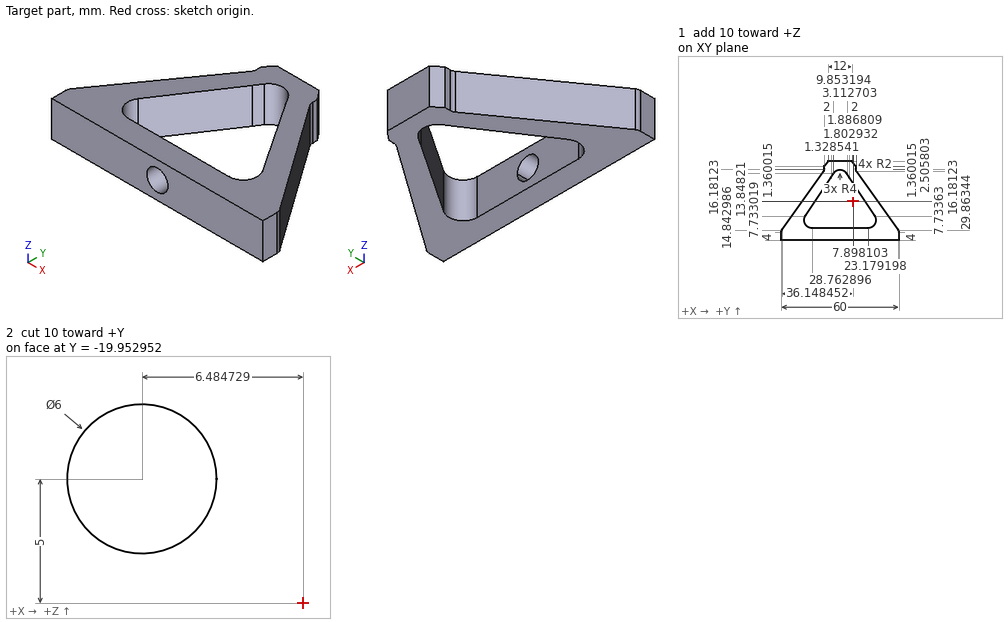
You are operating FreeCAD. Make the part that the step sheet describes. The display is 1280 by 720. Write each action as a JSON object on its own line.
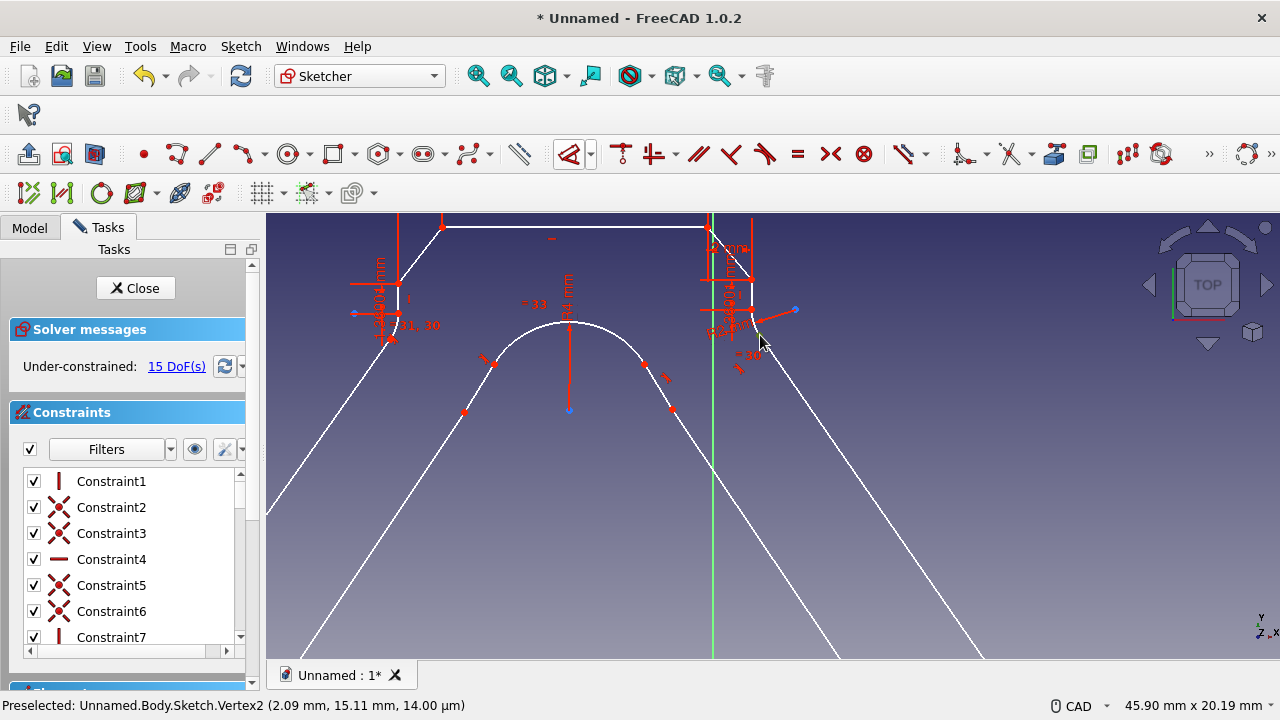
{"action": "left_click", "coordinate": [590, 154]}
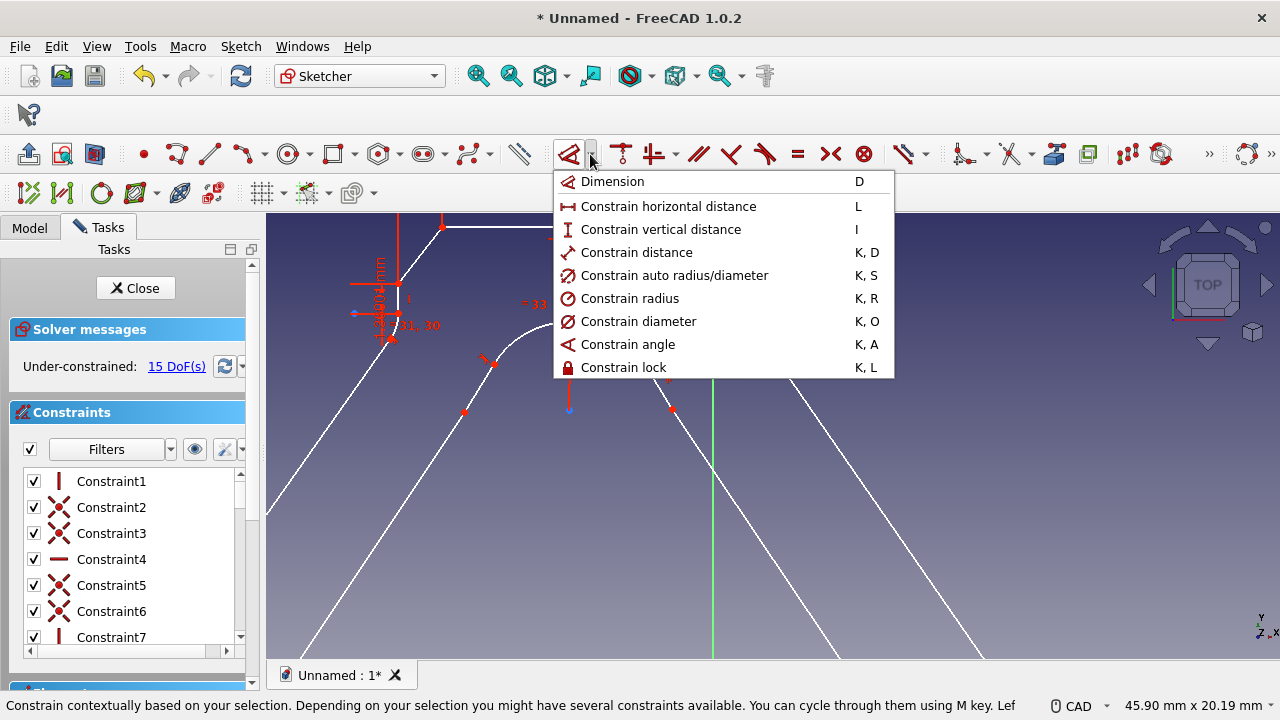
{"action": "left_click", "coordinate": [724, 206]}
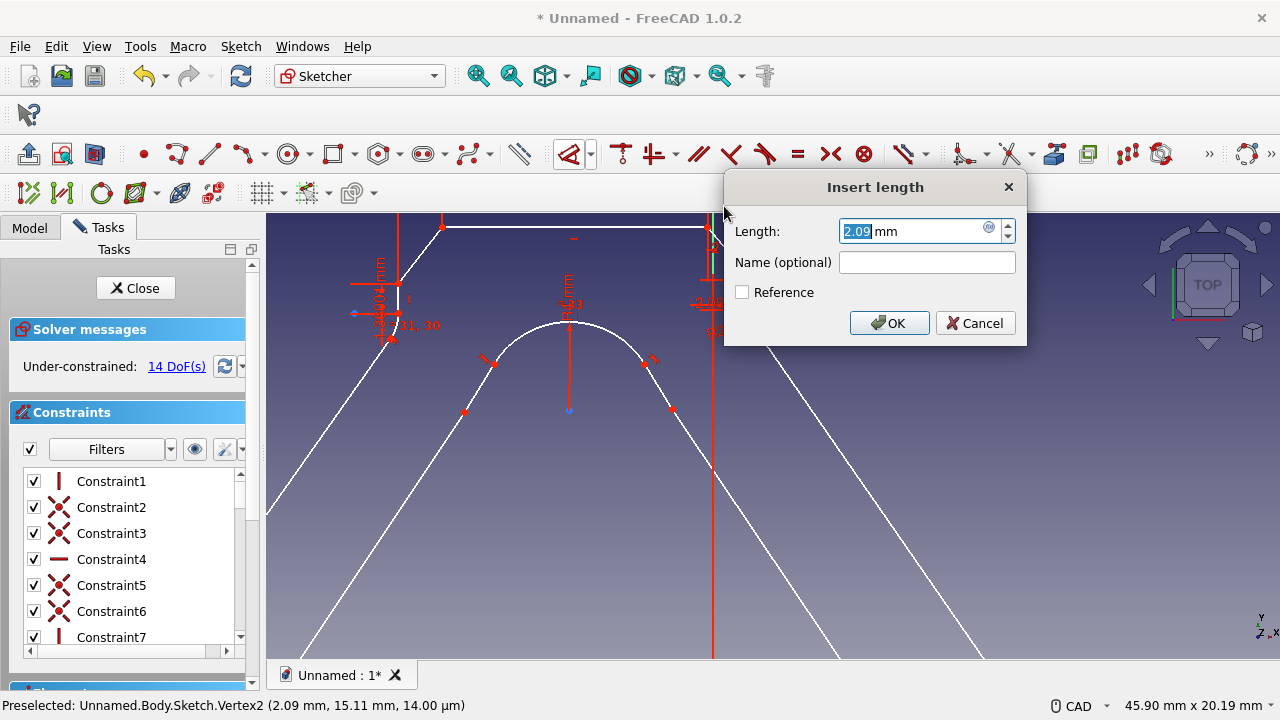
{"action": "type", "text": "1.886809"}
{"action": "key", "text": "Return"}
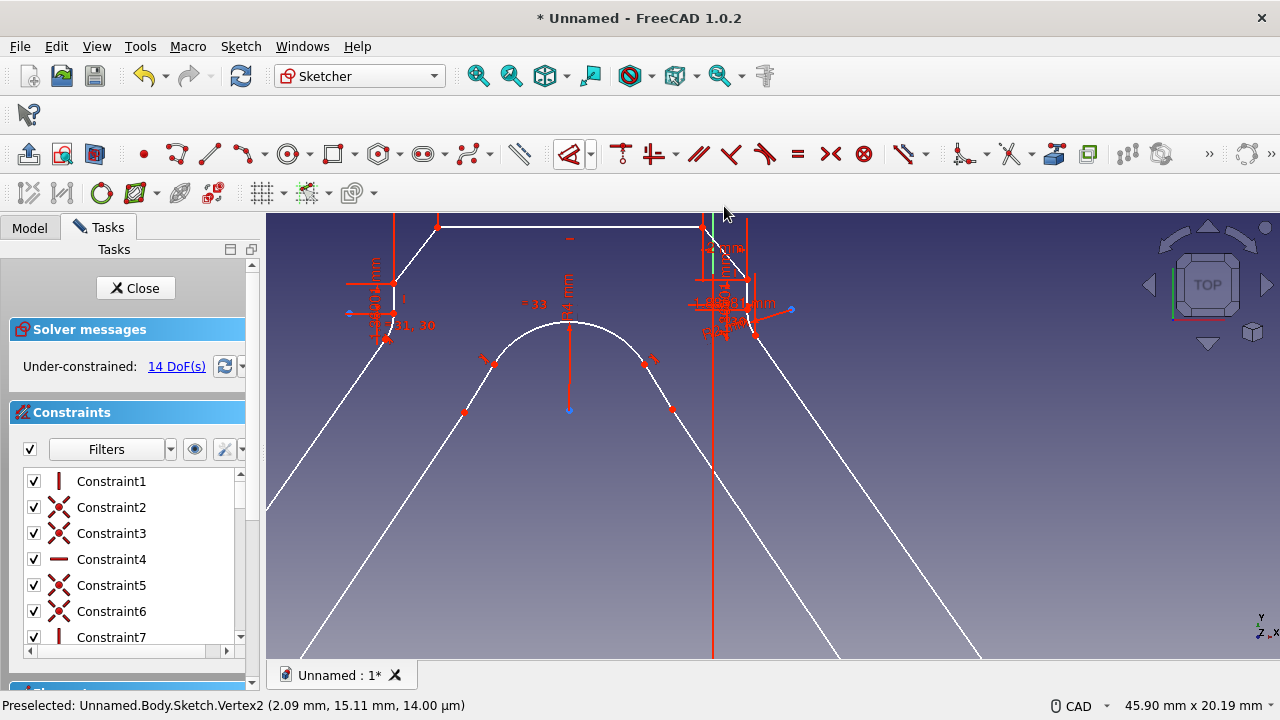
{"action": "left_click", "coordinate": [747, 310]}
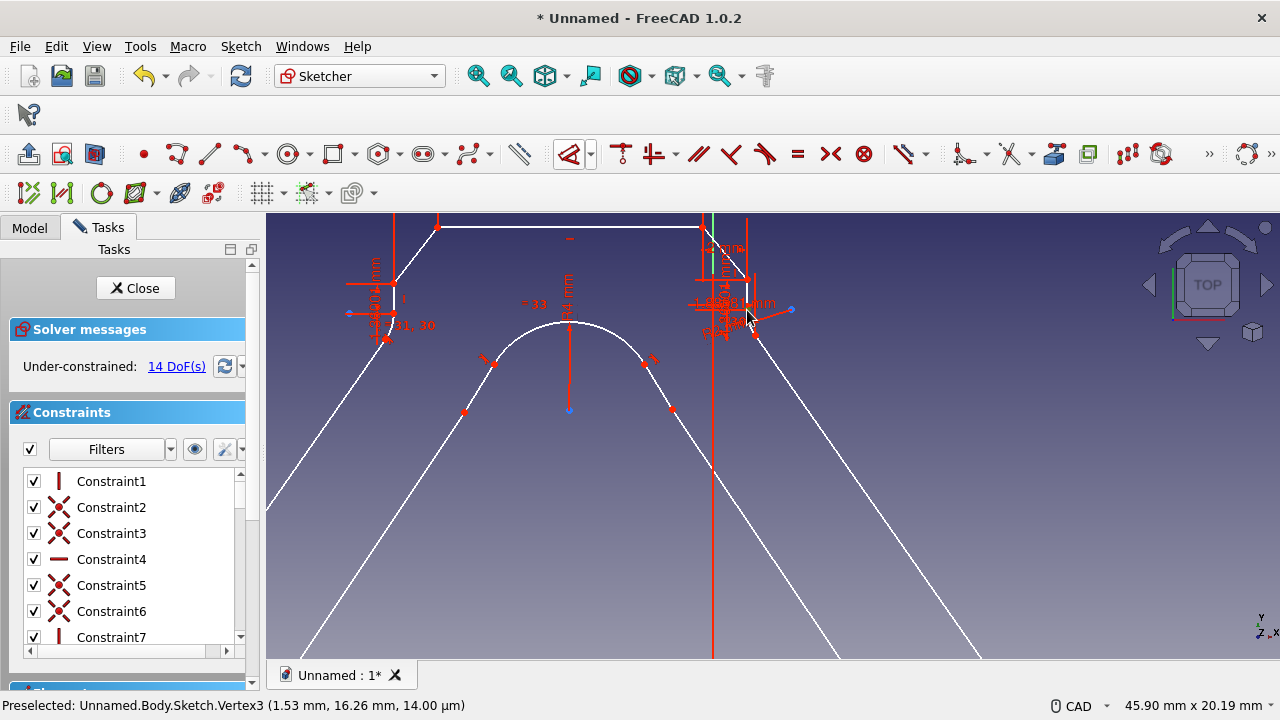
{"action": "key", "text": "i"}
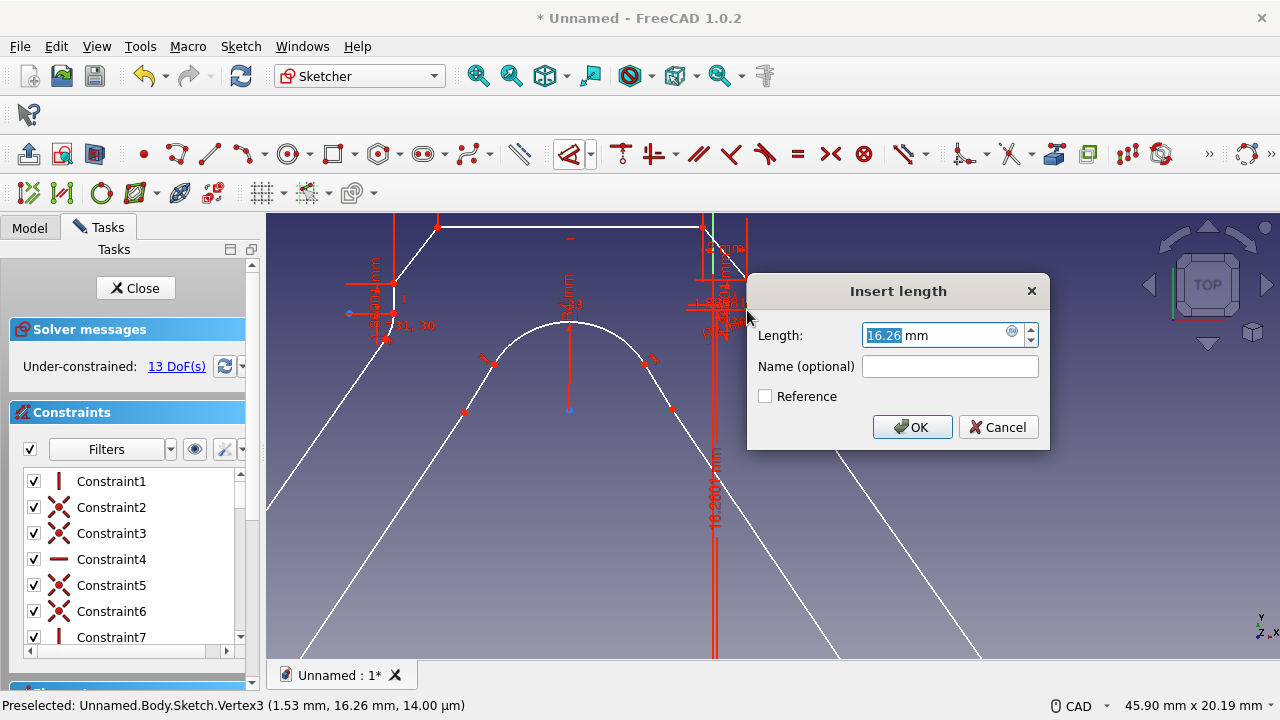
{"action": "type", "text": "16.18123"}
{"action": "key", "text": "Return"}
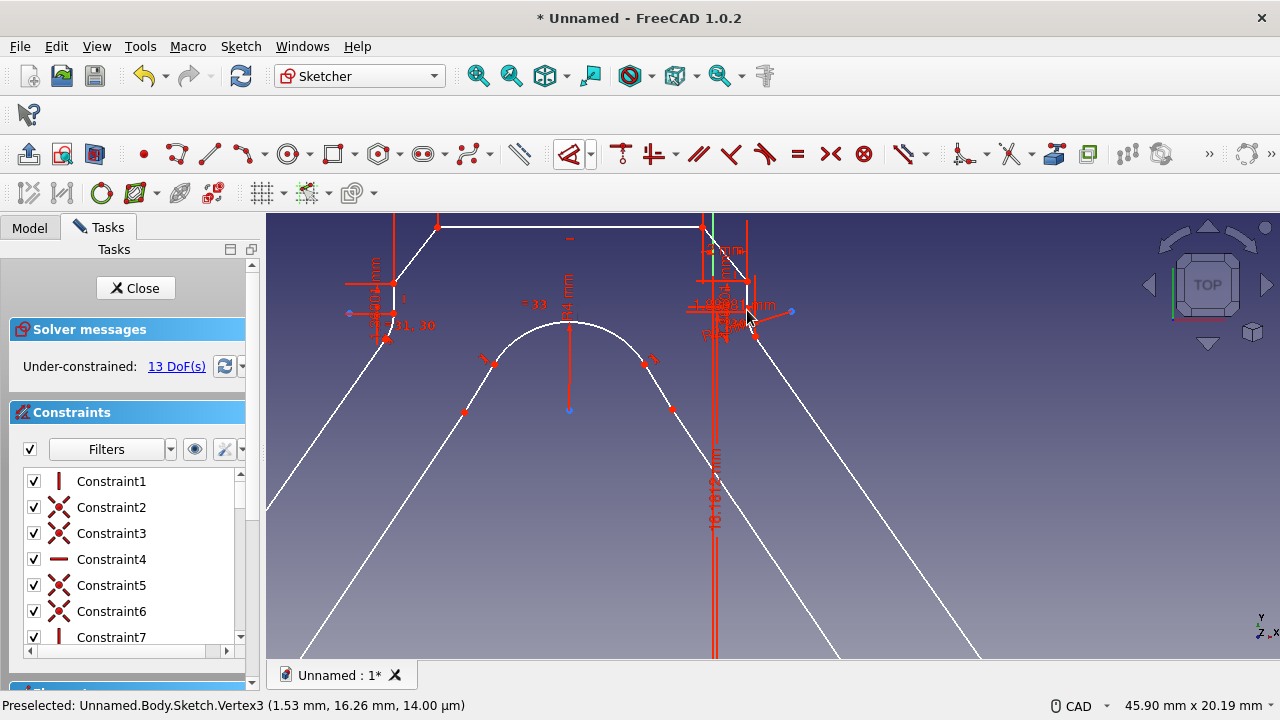
{"action": "left_click", "coordinate": [394, 314]}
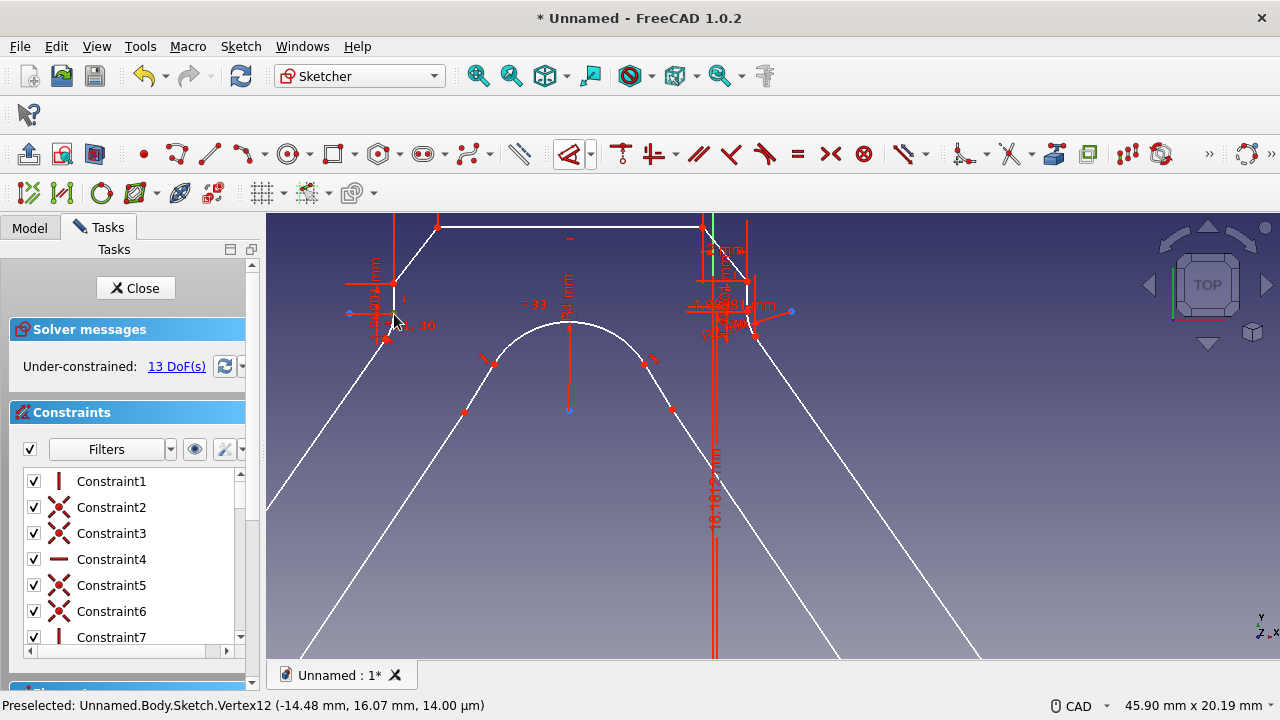
{"action": "left_click", "coordinate": [590, 154]}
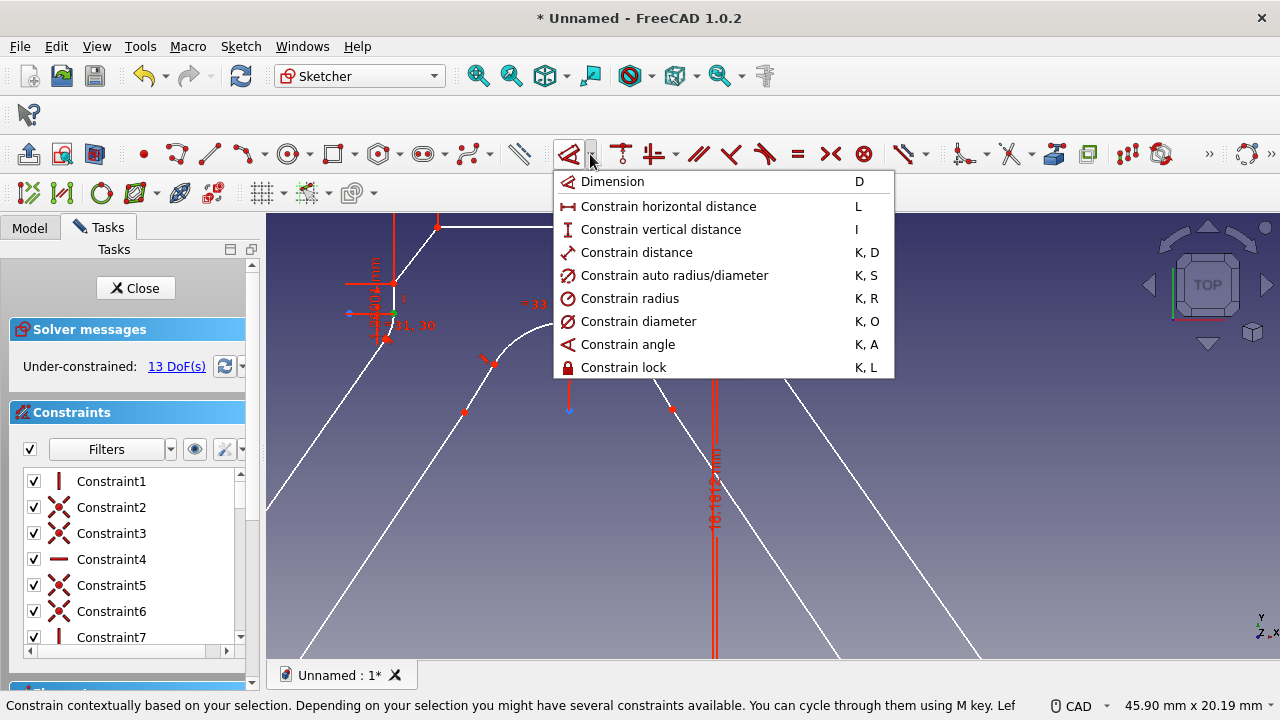
{"action": "left_click", "coordinate": [724, 230]}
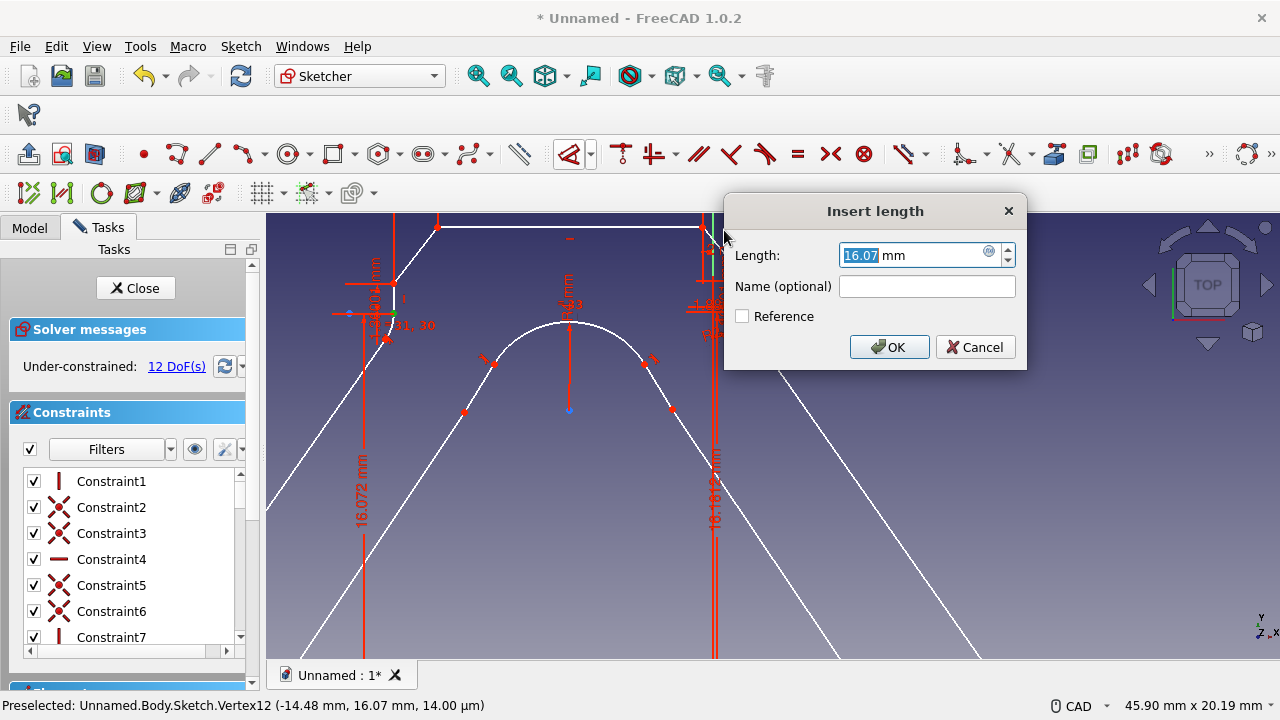
{"action": "type", "text": "16.18123"}
{"action": "key", "text": "Return"}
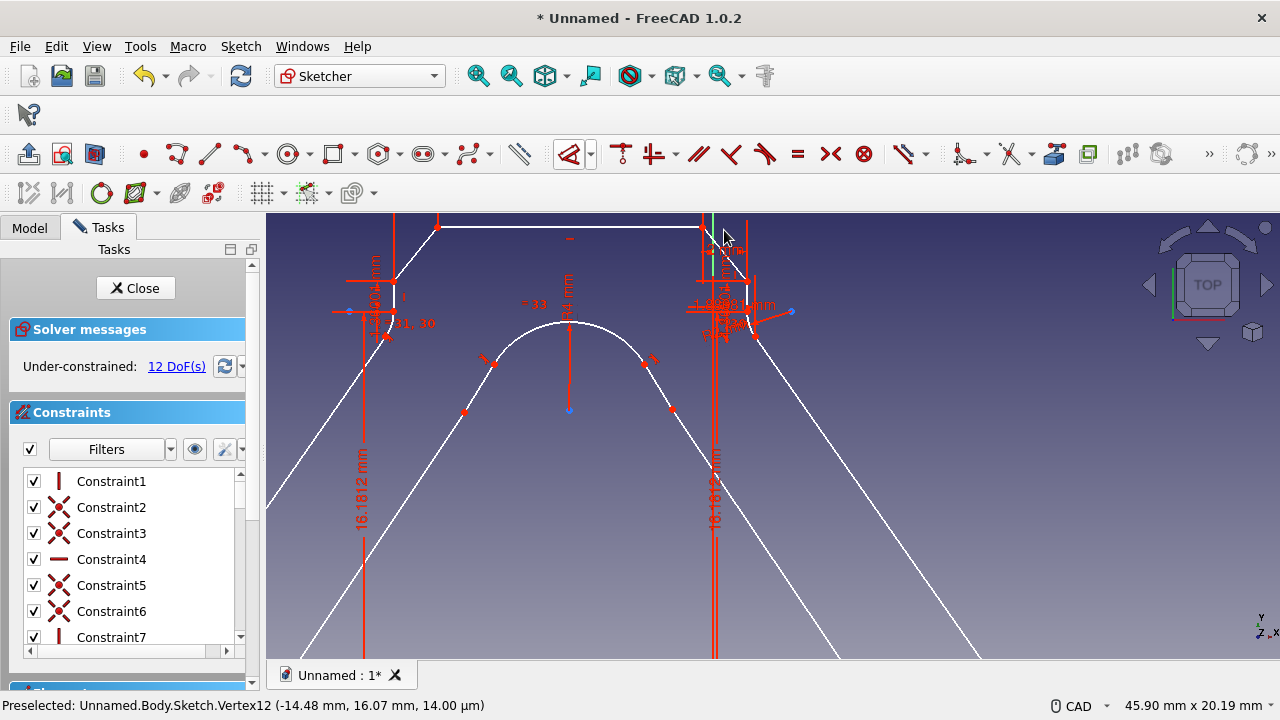
{"action": "scroll", "coordinate": [762, 336], "scroll_direction": "down", "scroll_amount": 6}